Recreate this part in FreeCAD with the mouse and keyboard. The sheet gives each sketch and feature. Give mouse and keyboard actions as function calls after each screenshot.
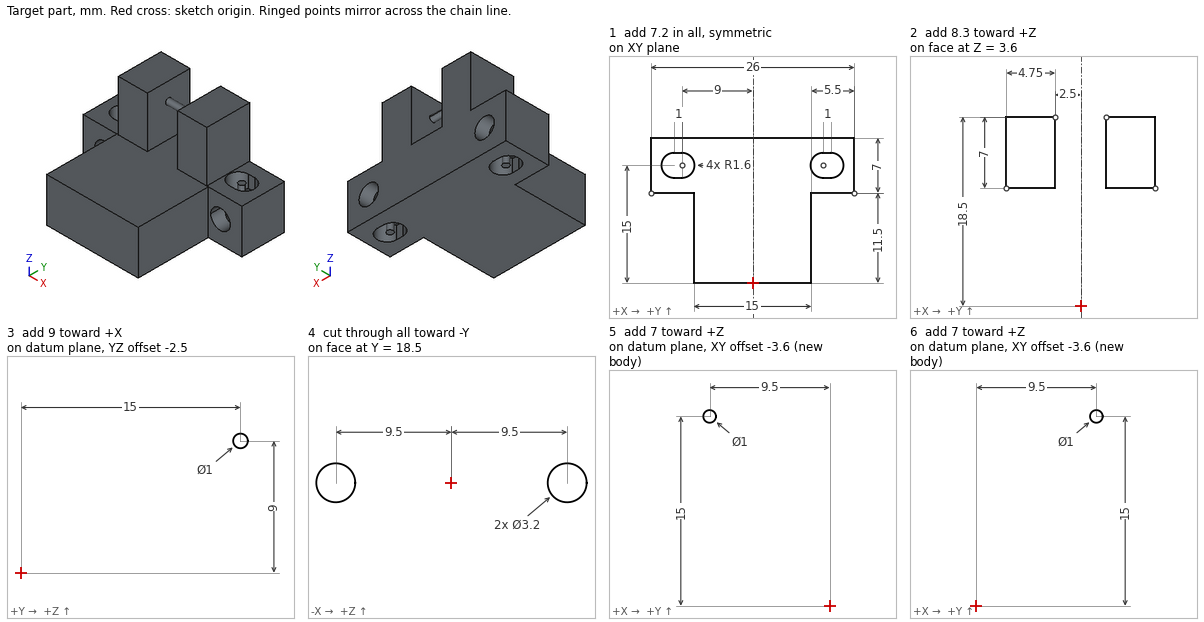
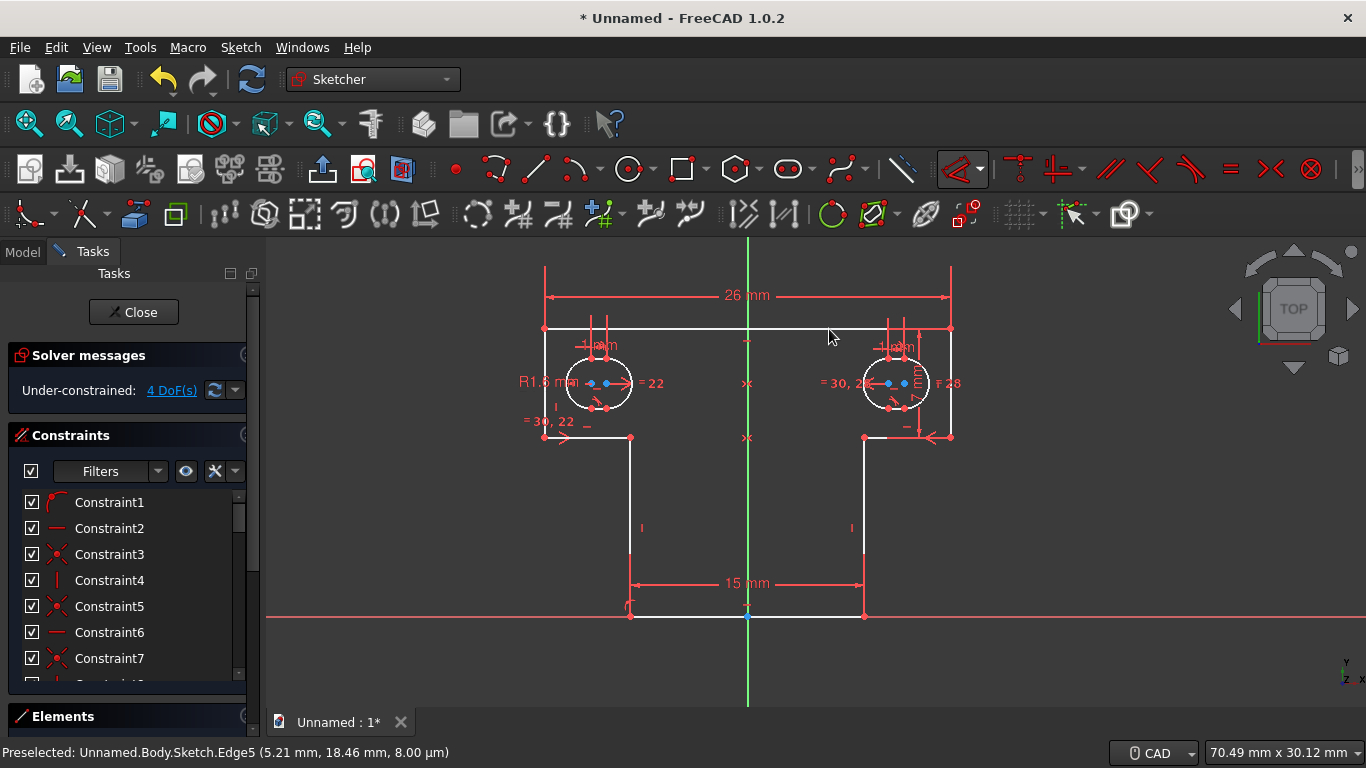
click(607, 409)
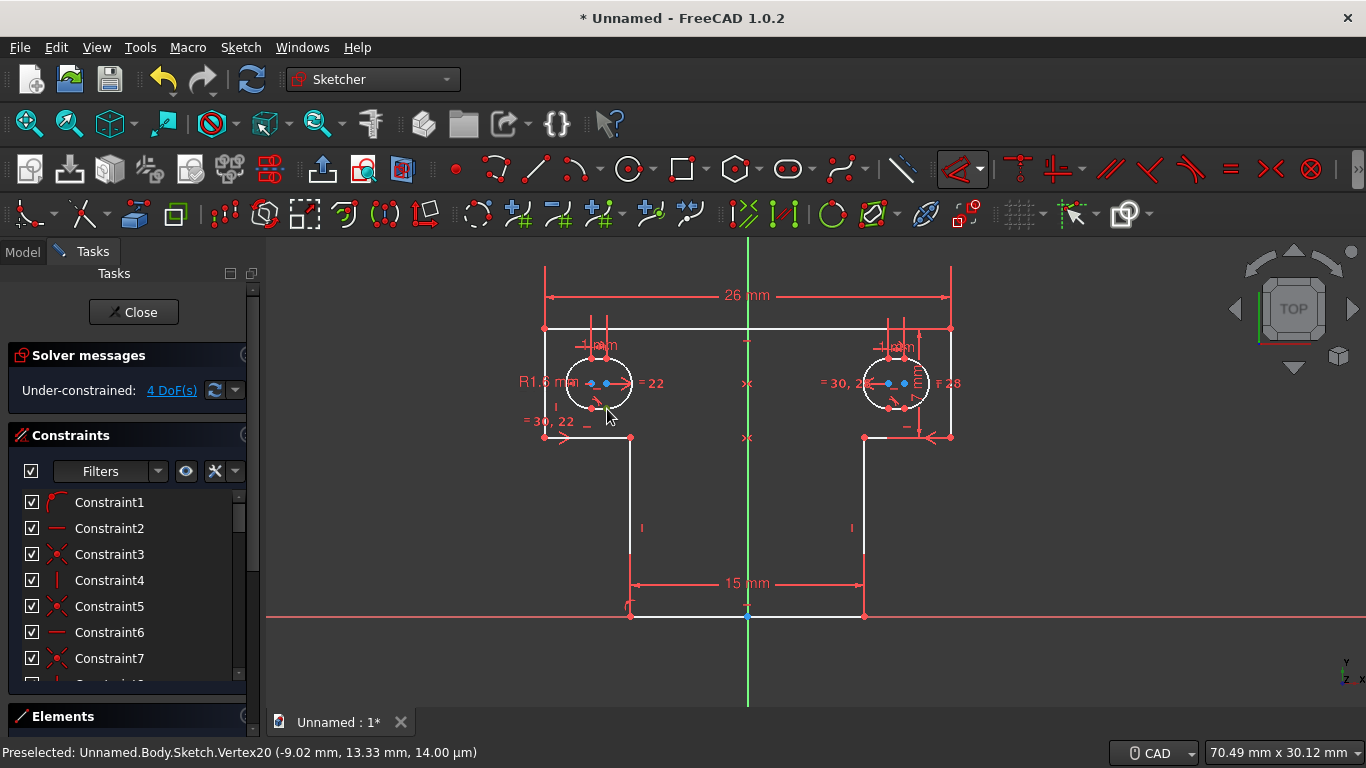
key(l)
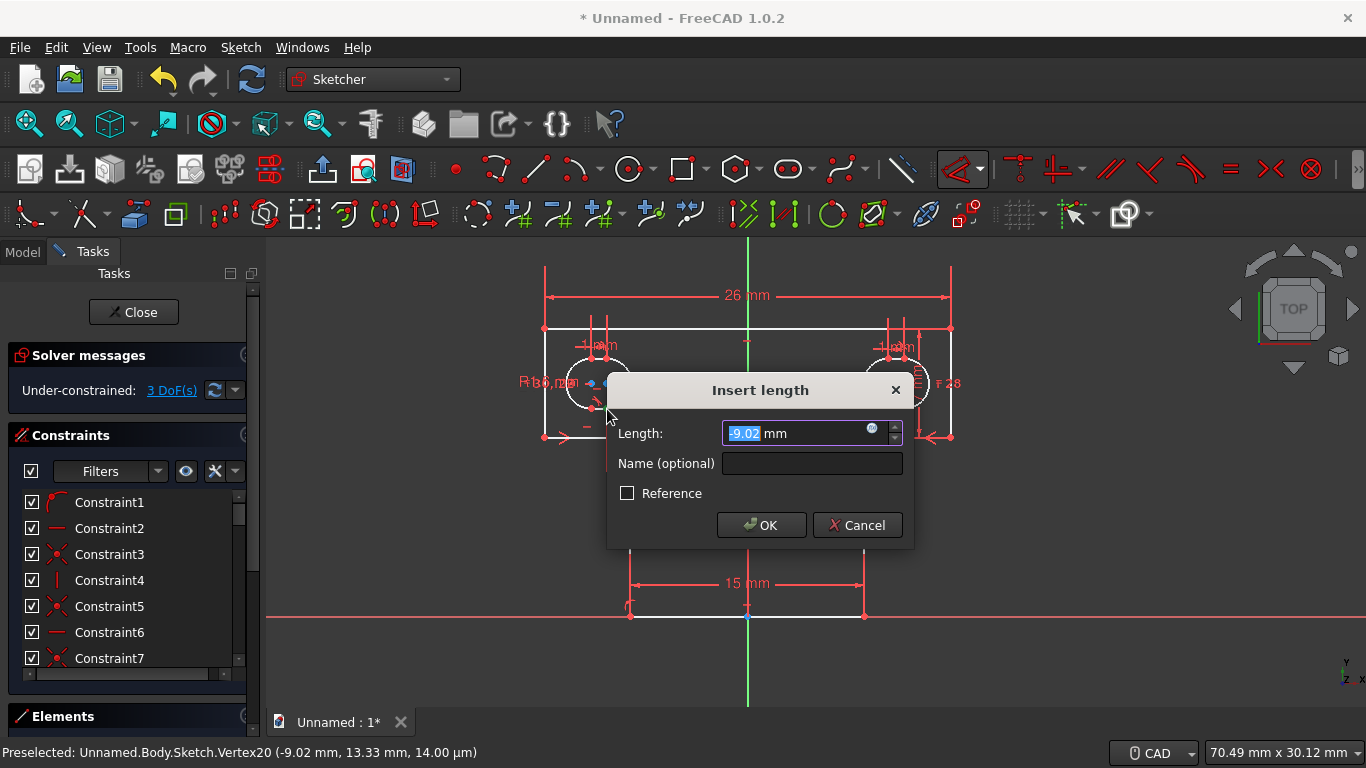
text(-9)
key(Return)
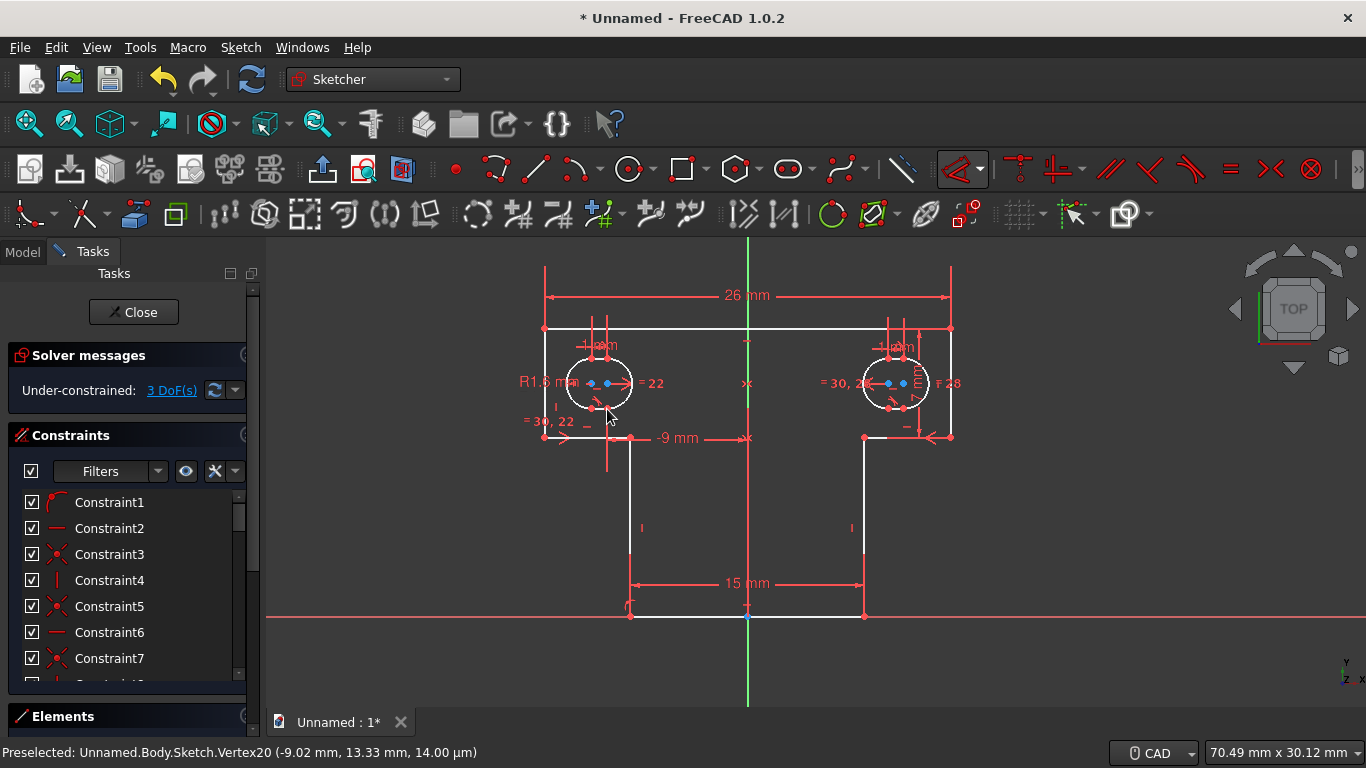
click(890, 438)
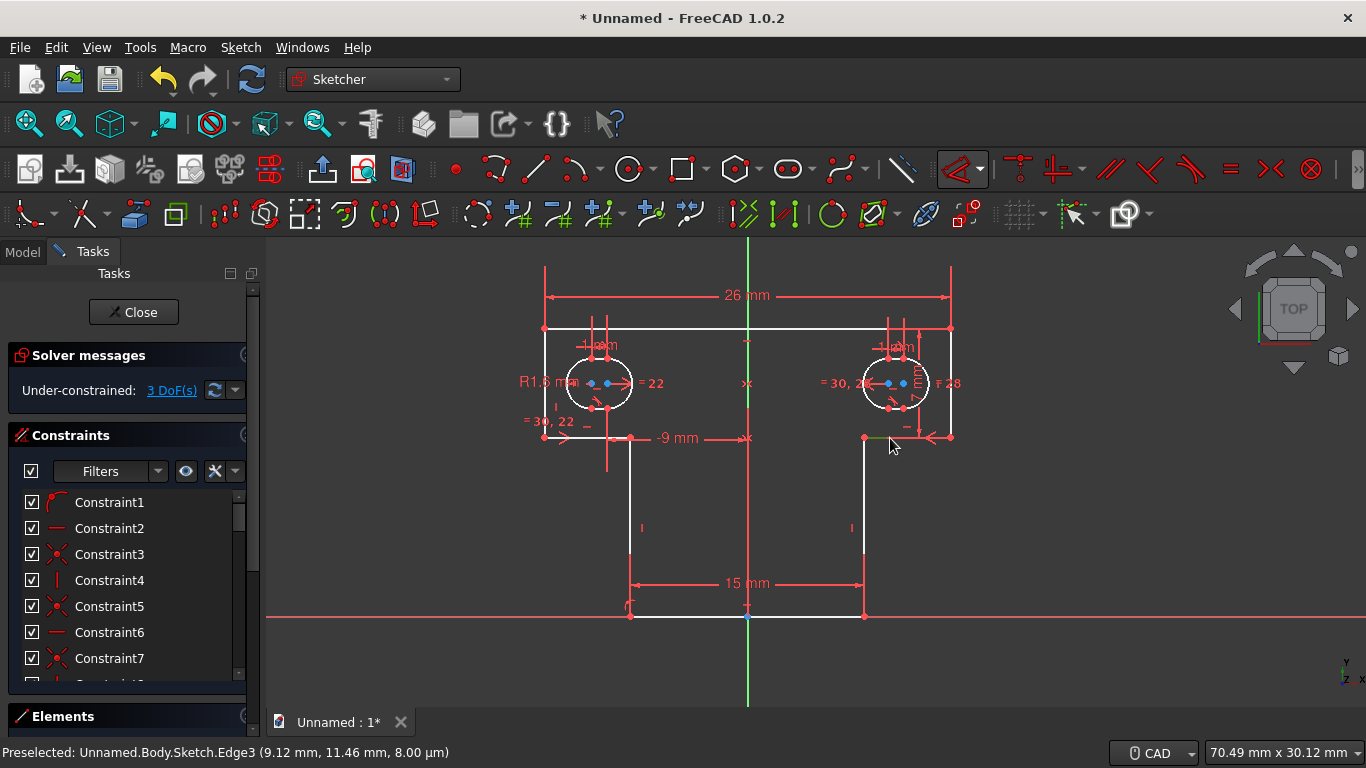
click(982, 170)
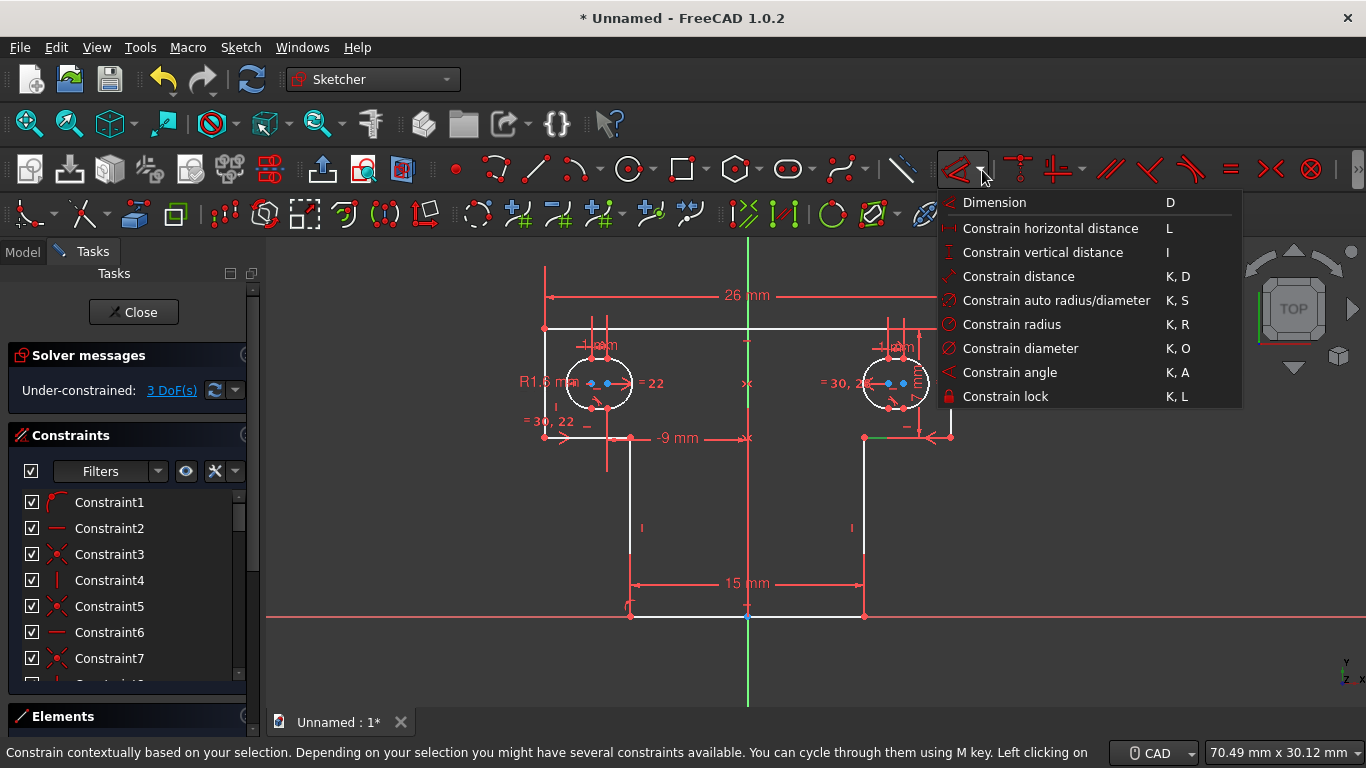
click(1090, 228)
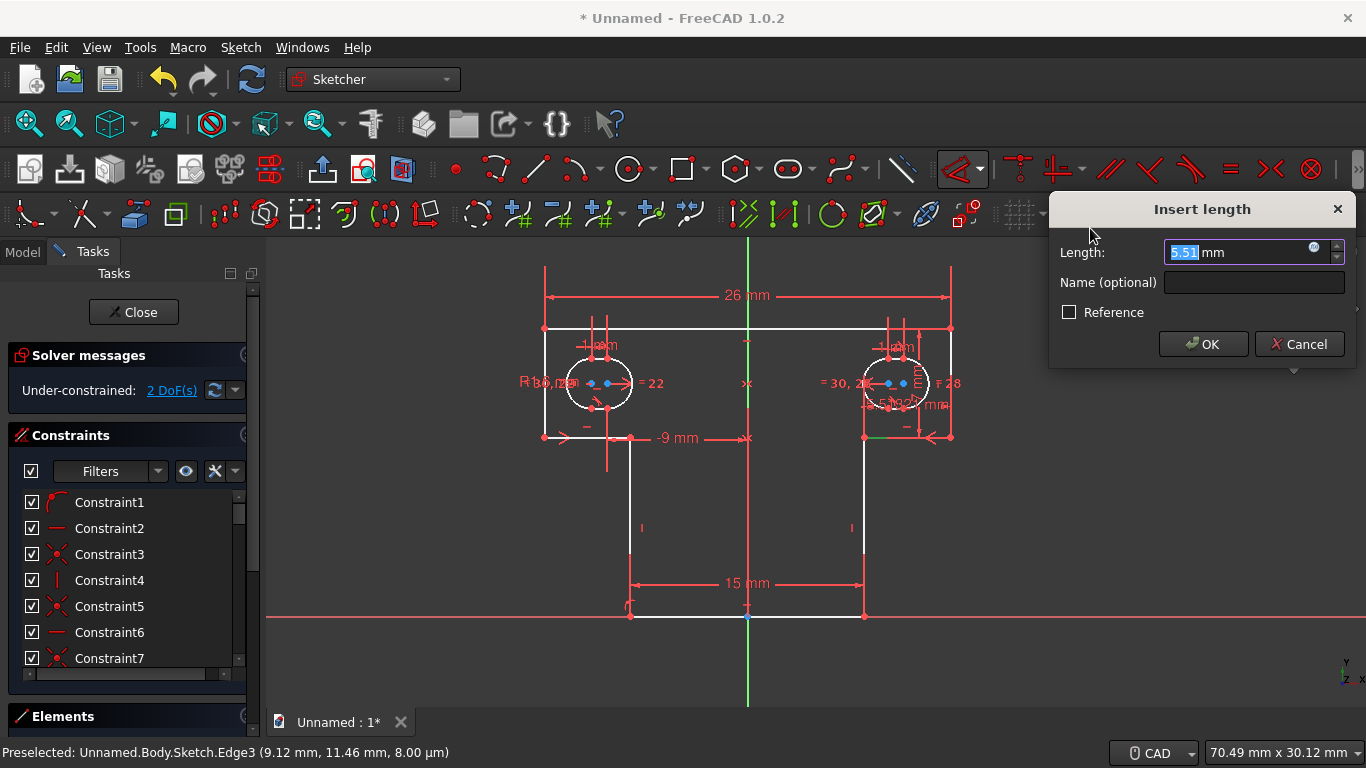
text(5.5)
key(Return)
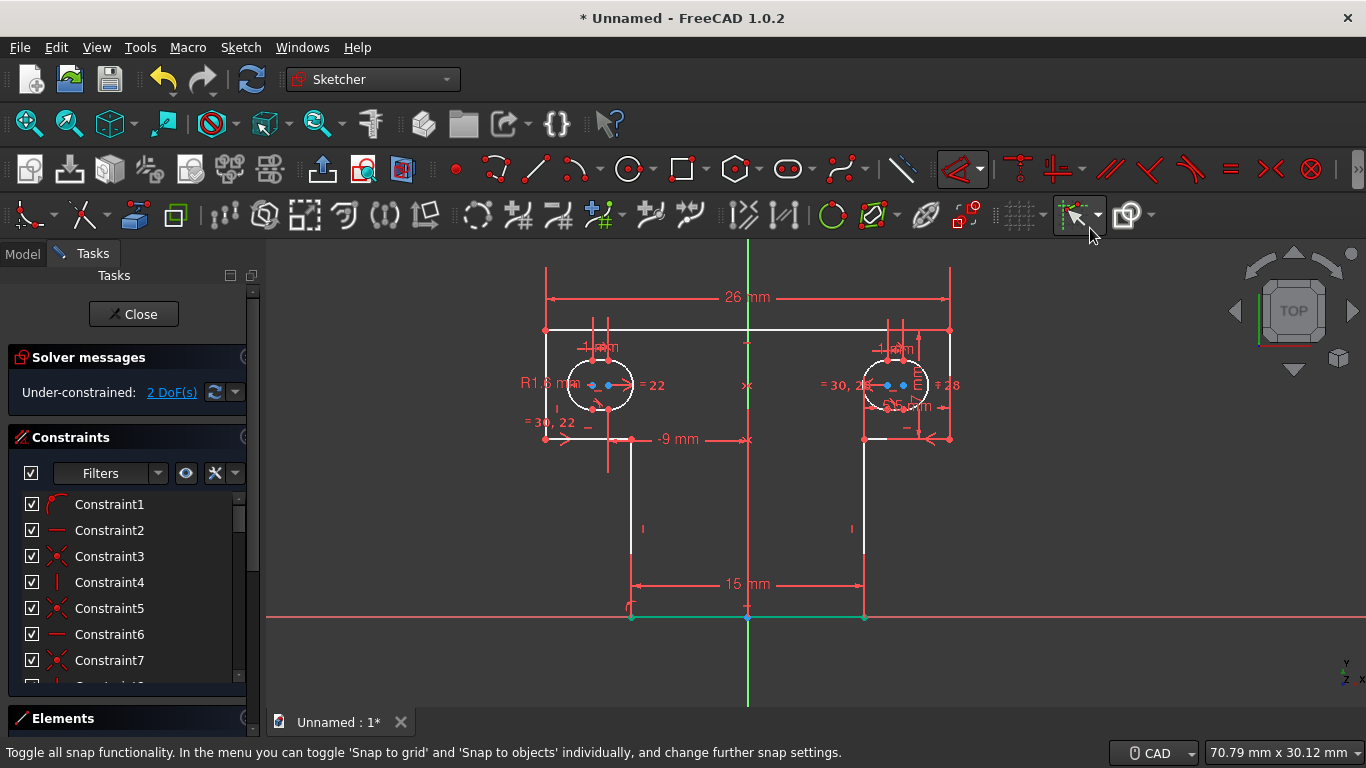
click(593, 385)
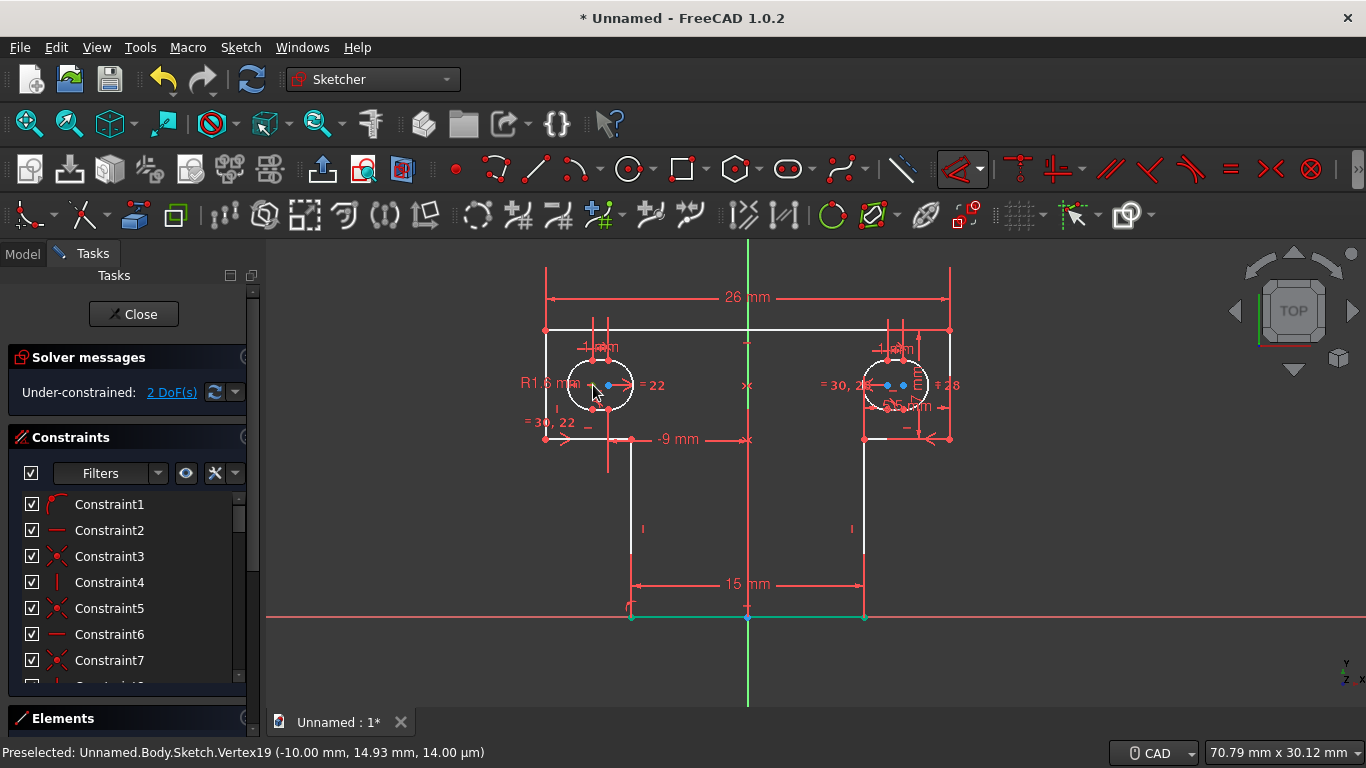
key(i)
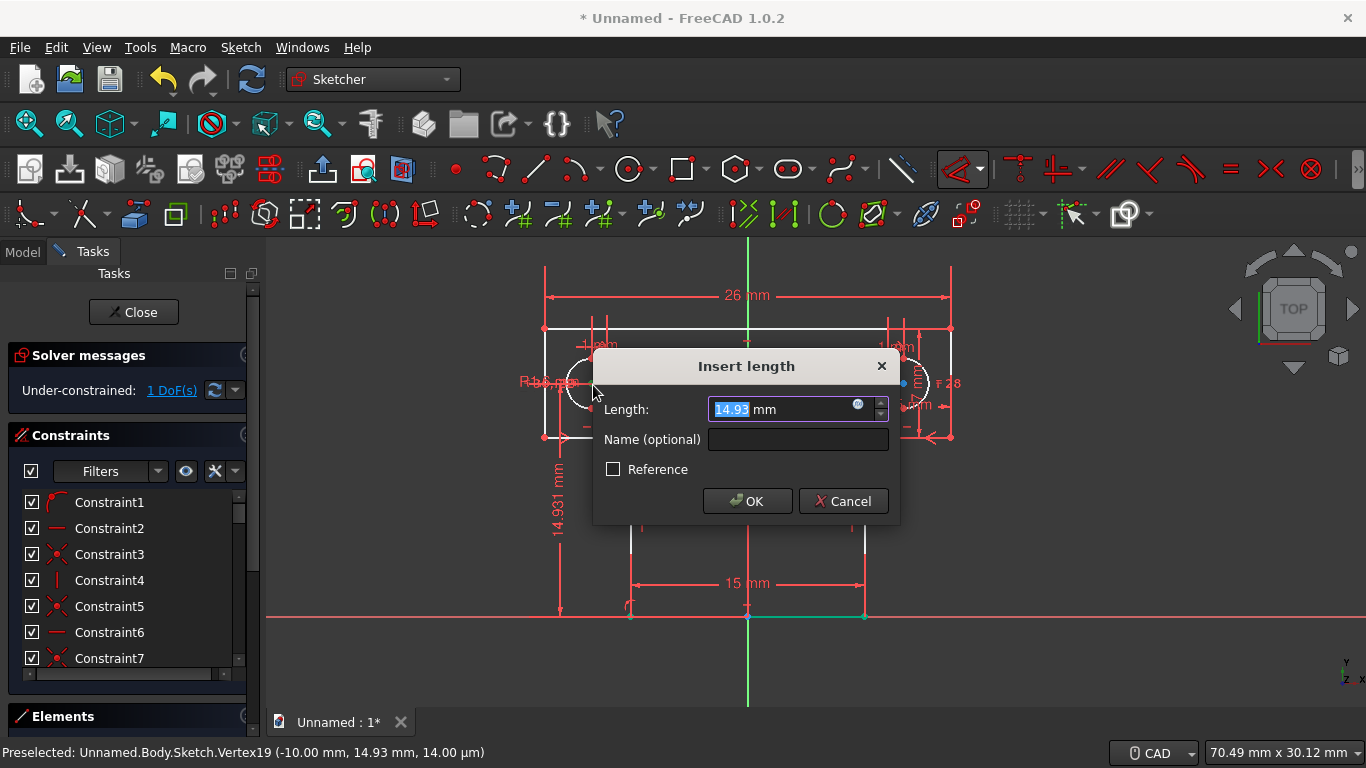
text(15)
key(Return)